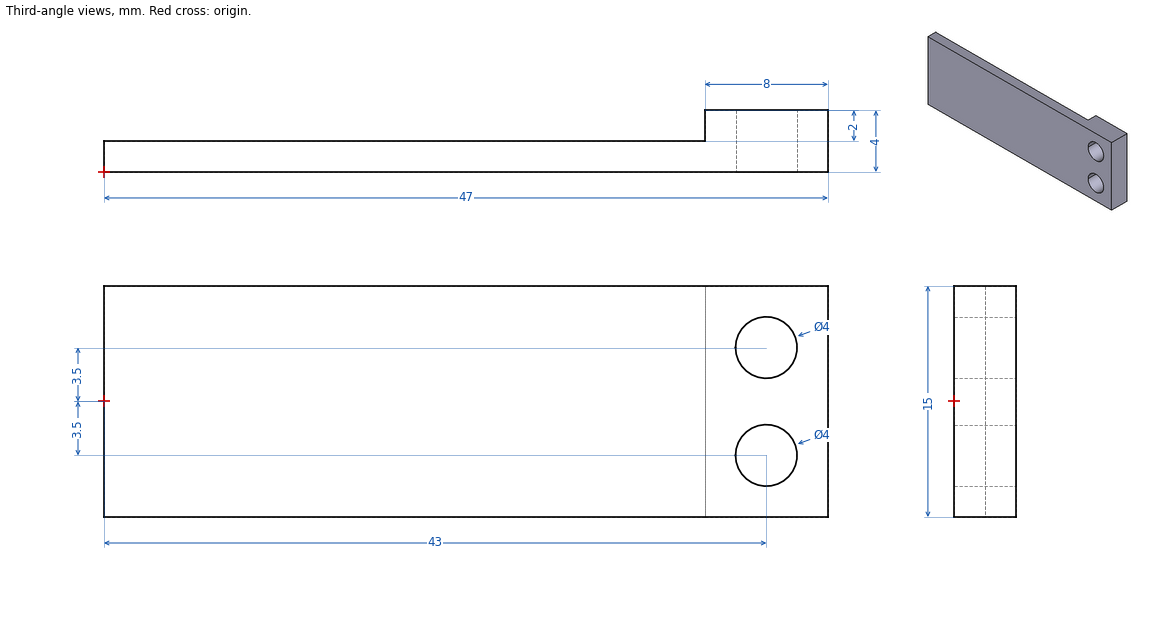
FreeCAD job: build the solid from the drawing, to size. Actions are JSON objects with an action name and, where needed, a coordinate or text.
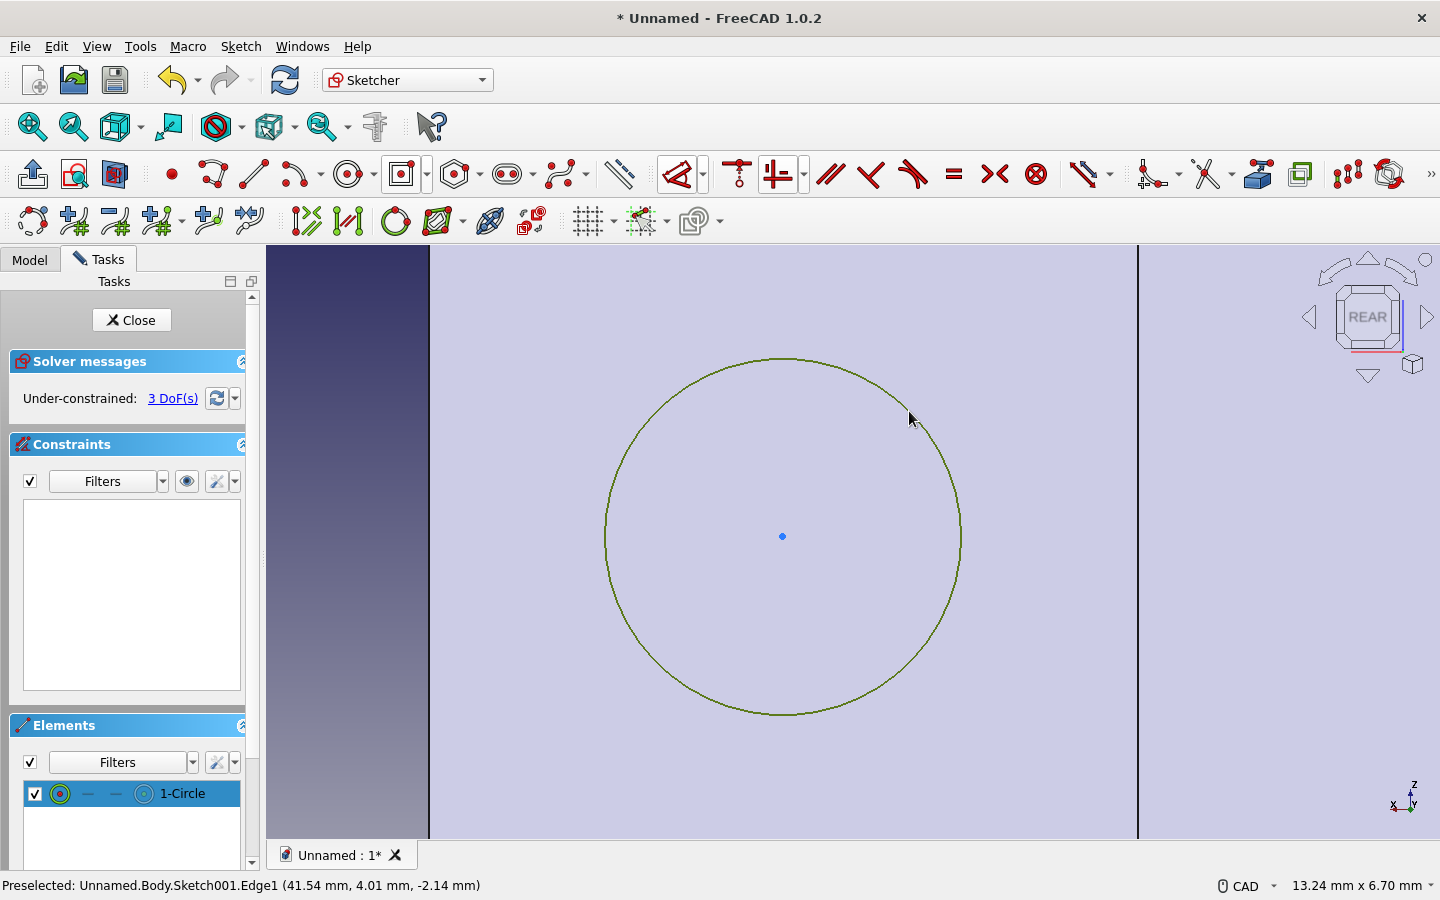
{"action": "left_click", "coordinate": [702, 174]}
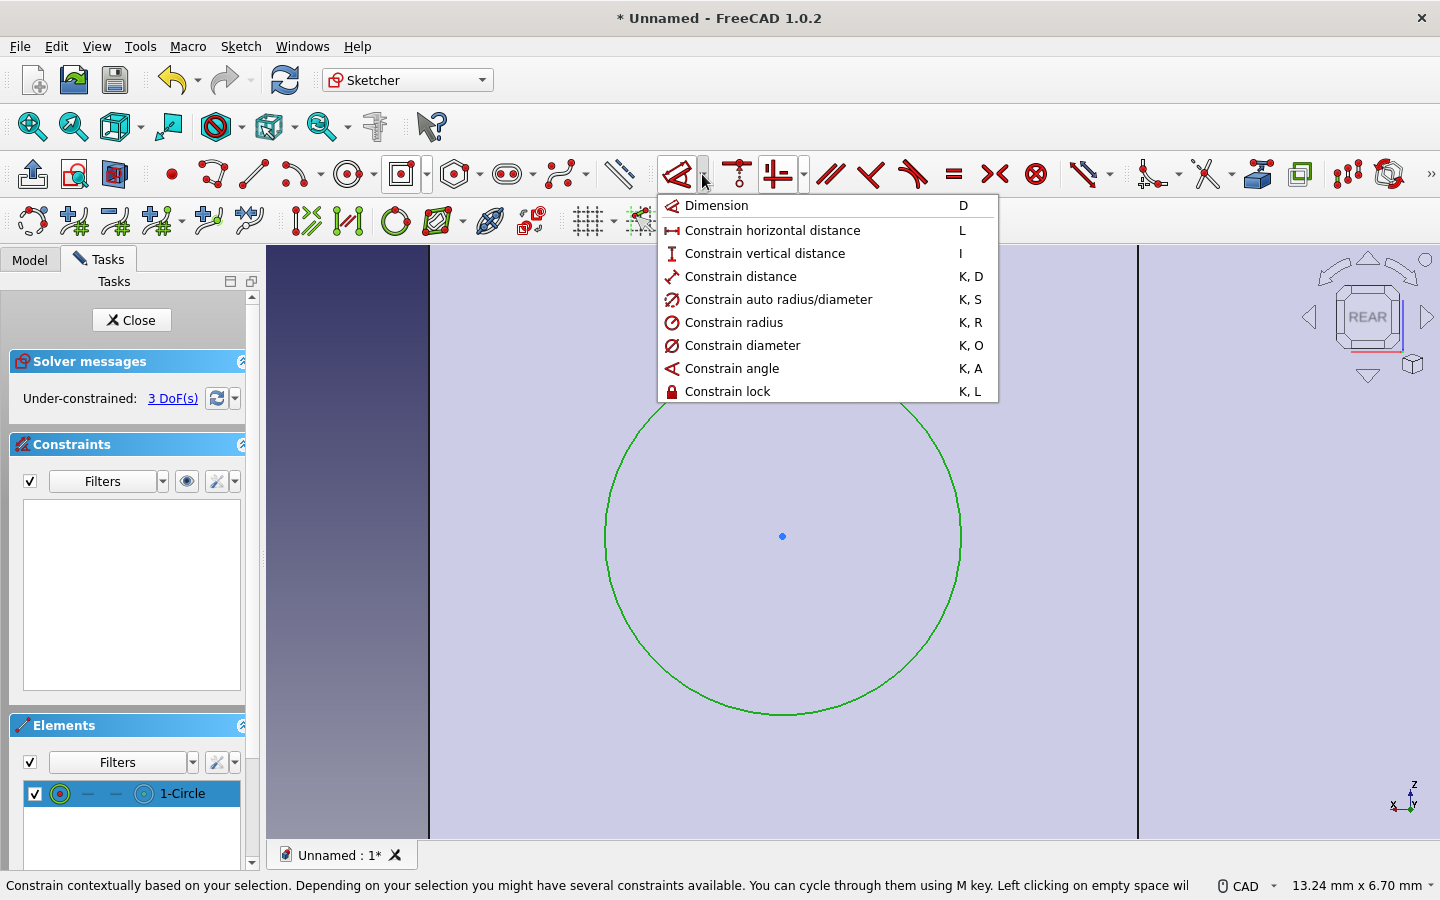
{"action": "left_click", "coordinate": [828, 346]}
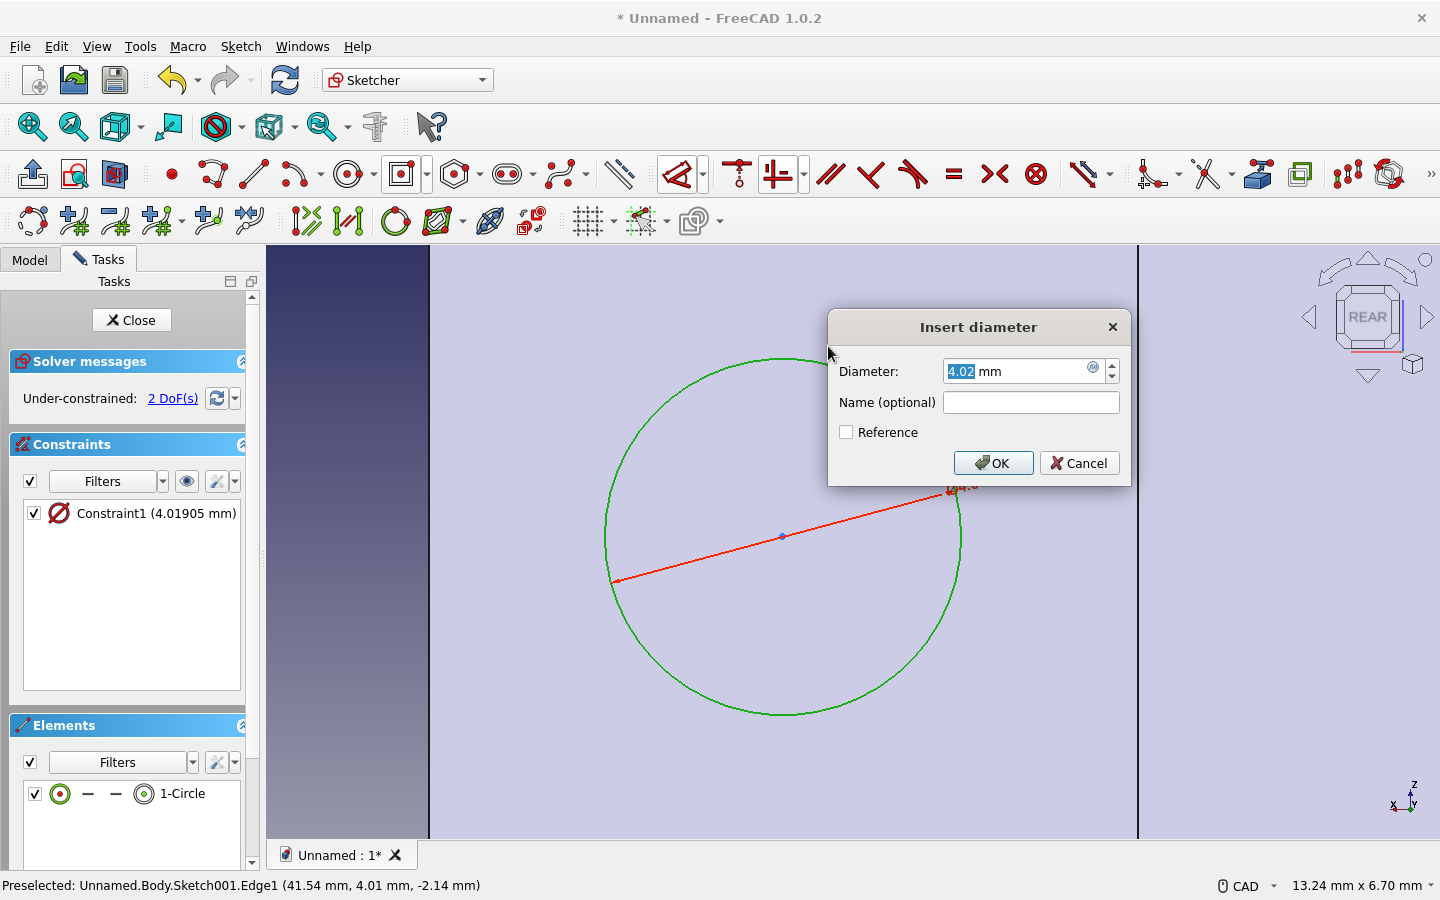
{"action": "type", "text": "4"}
{"action": "key", "text": "Return"}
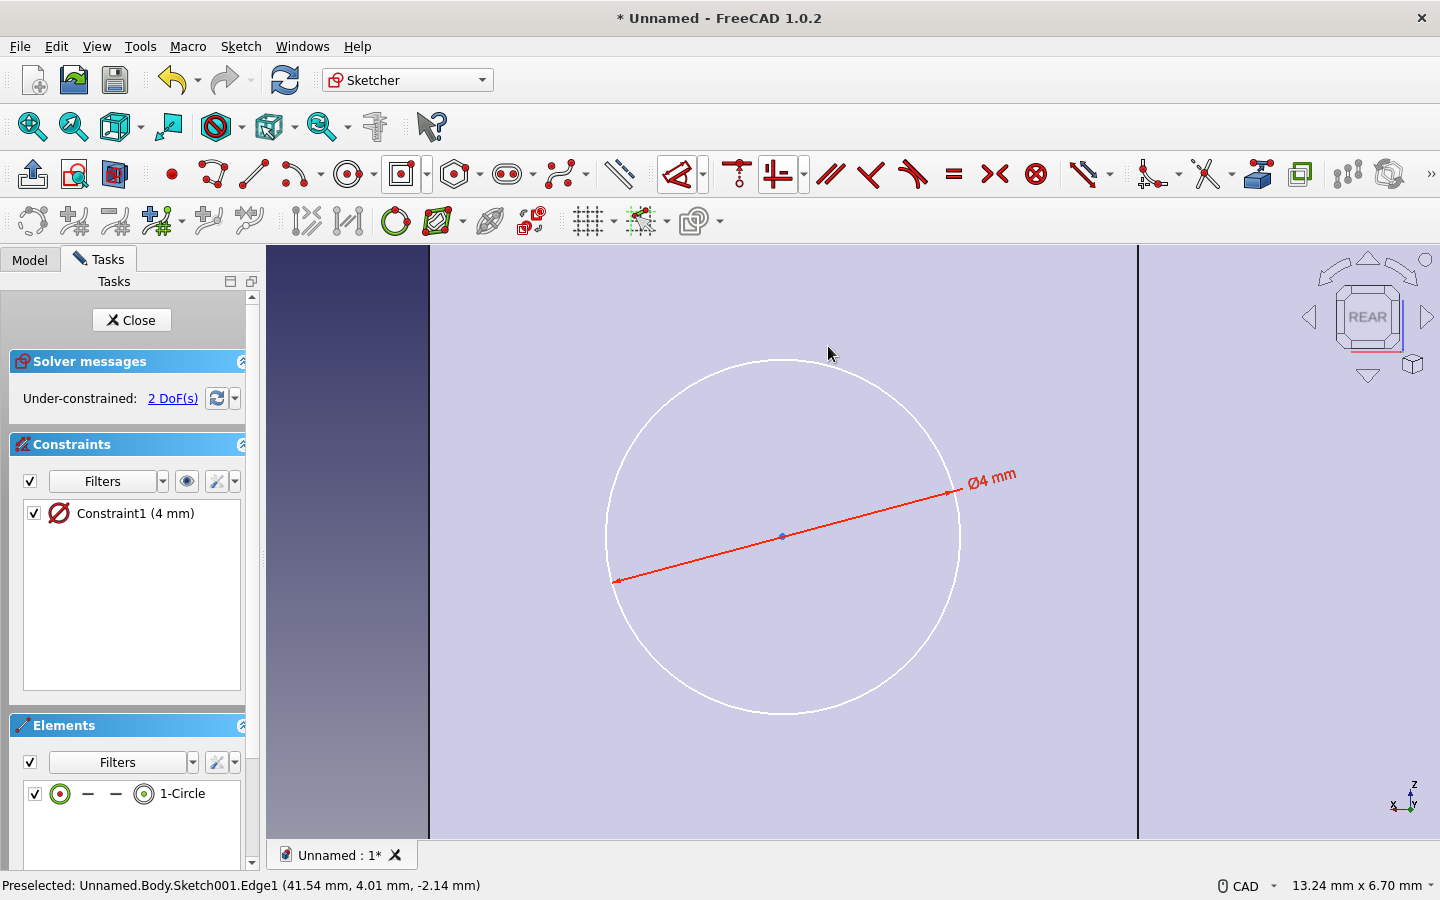
{"action": "left_click", "coordinate": [783, 537]}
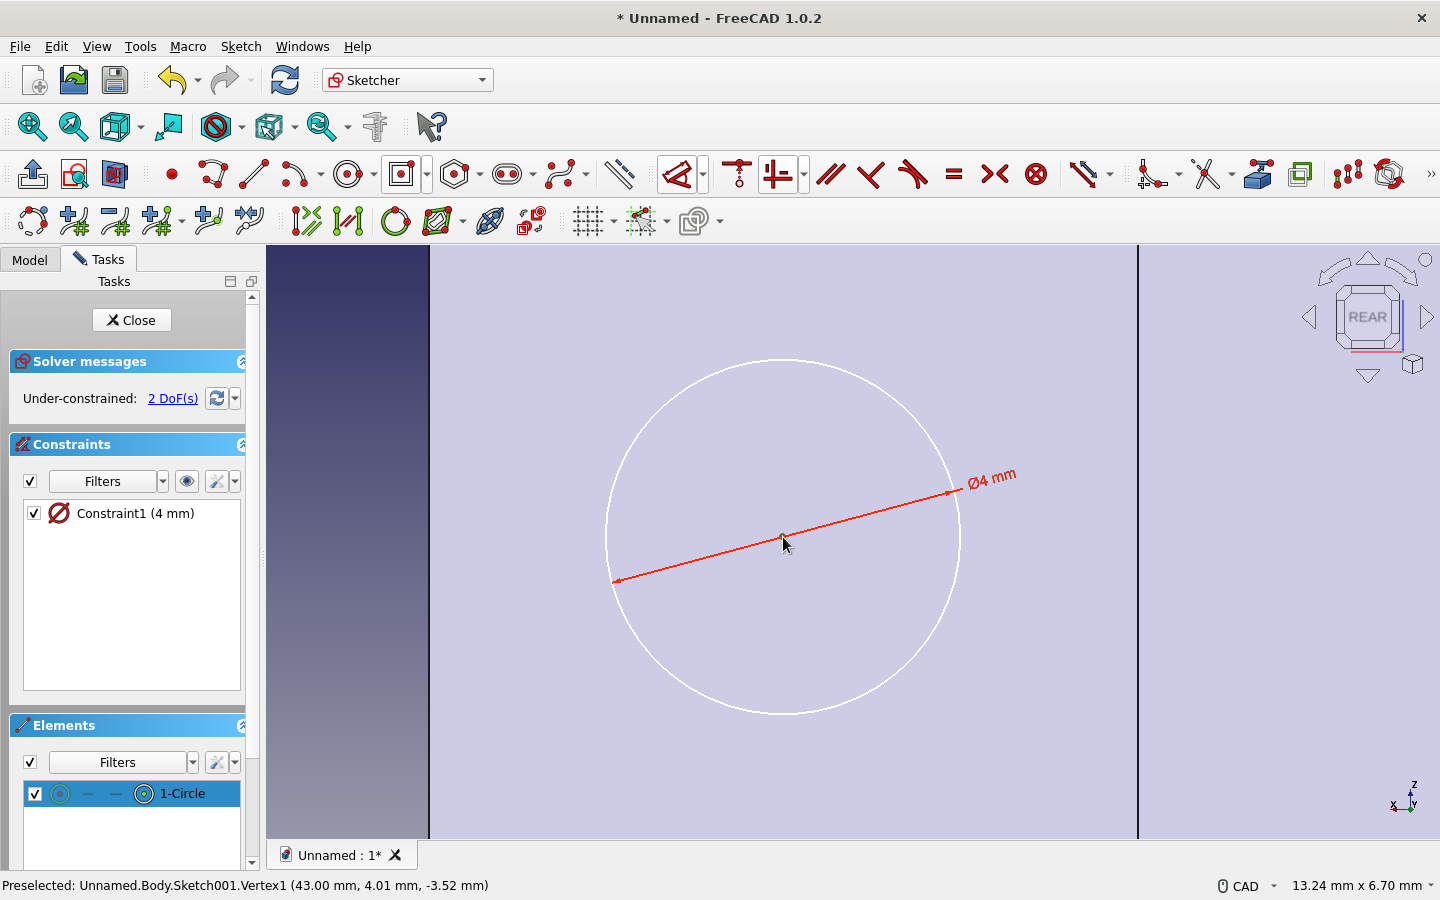
{"action": "left_click", "coordinate": [702, 174]}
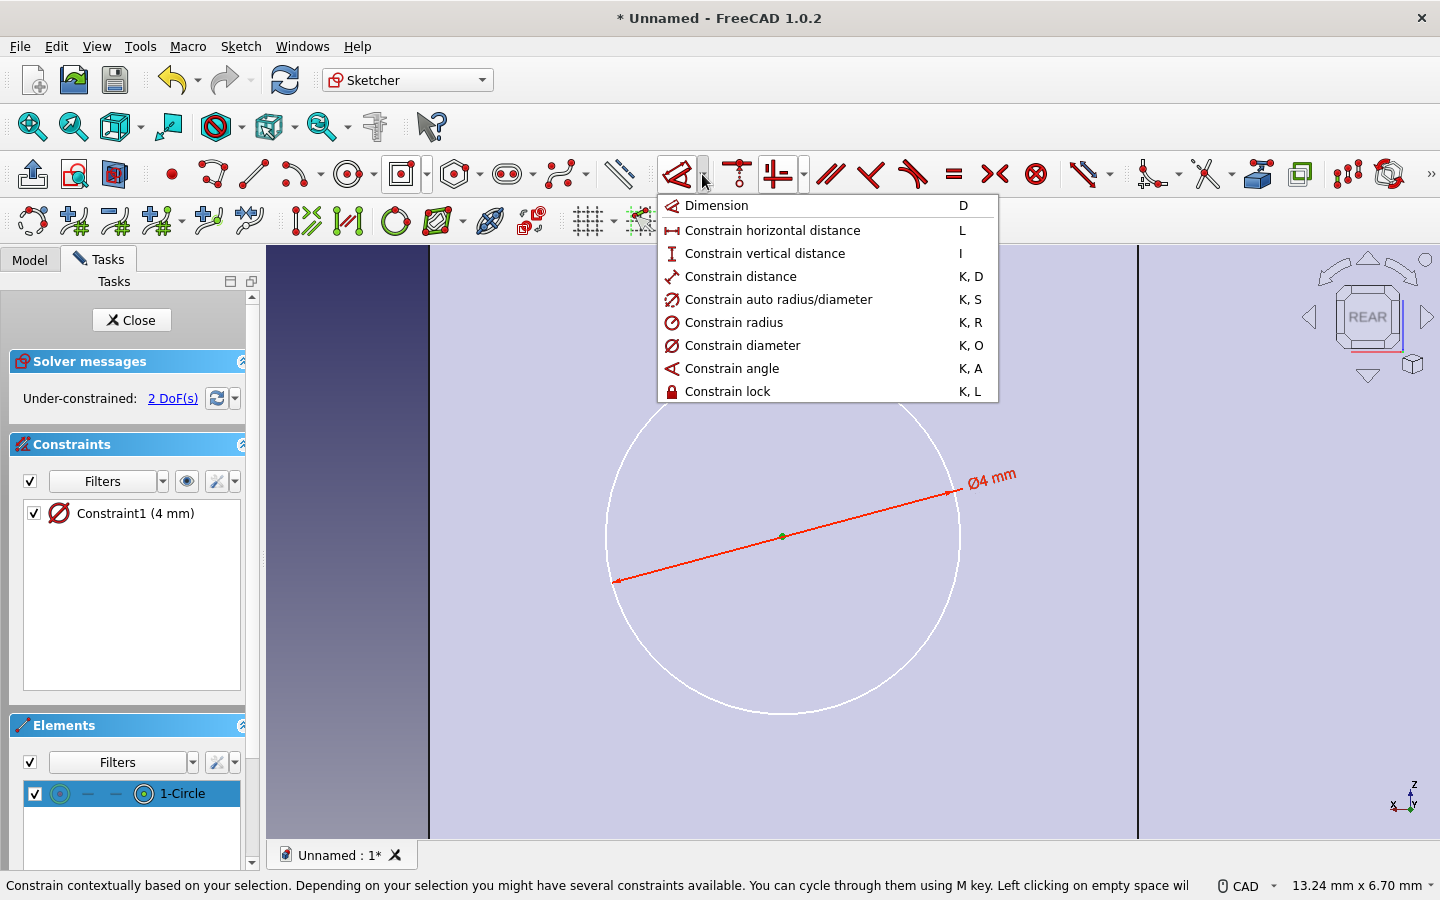
{"action": "left_click", "coordinate": [828, 230]}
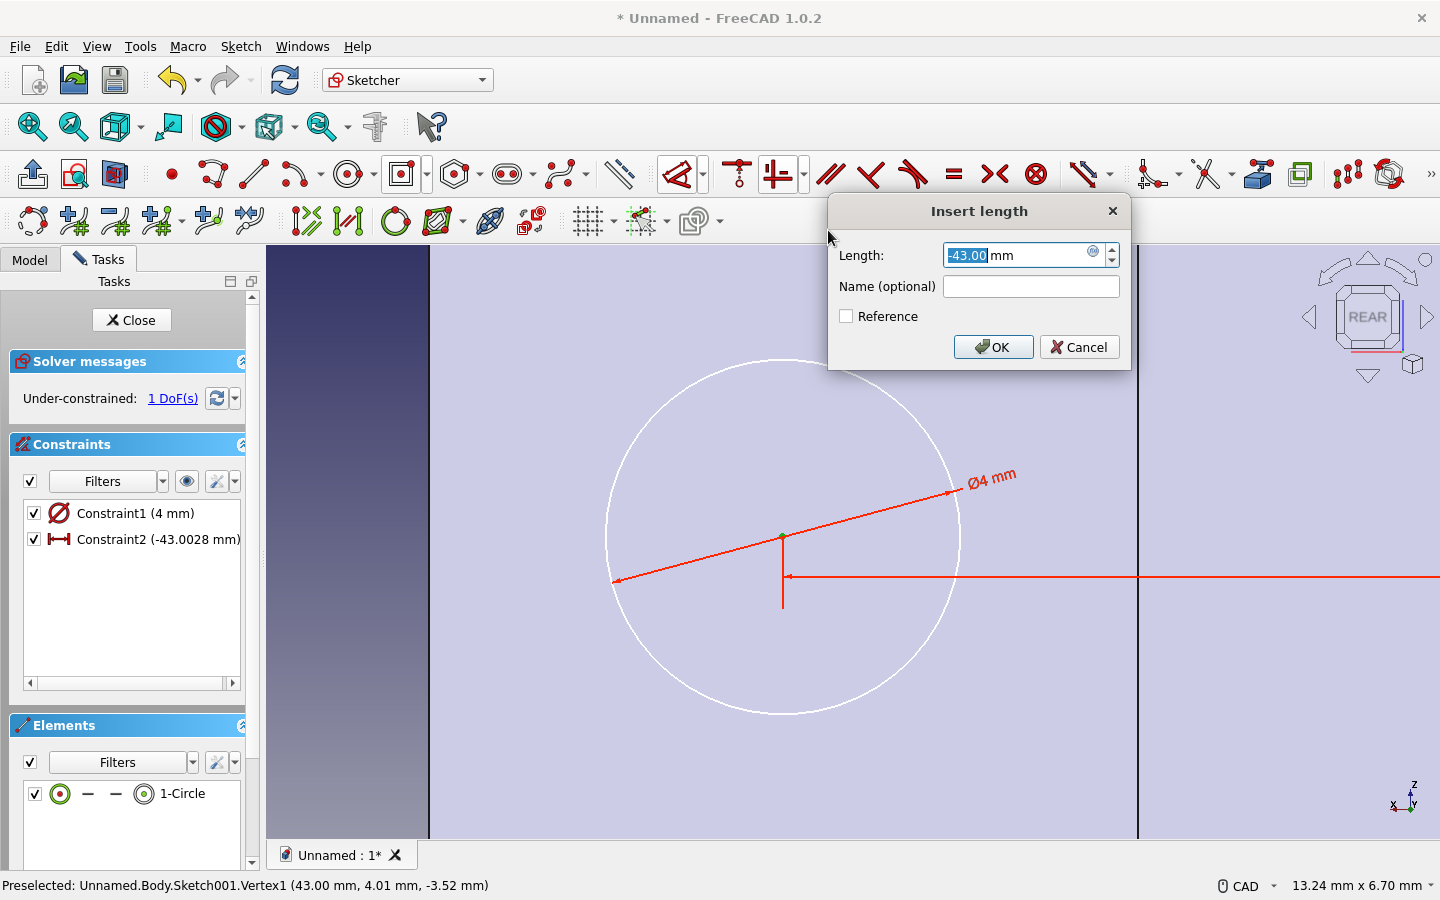
{"action": "type", "text": "-43"}
{"action": "key", "text": "Return"}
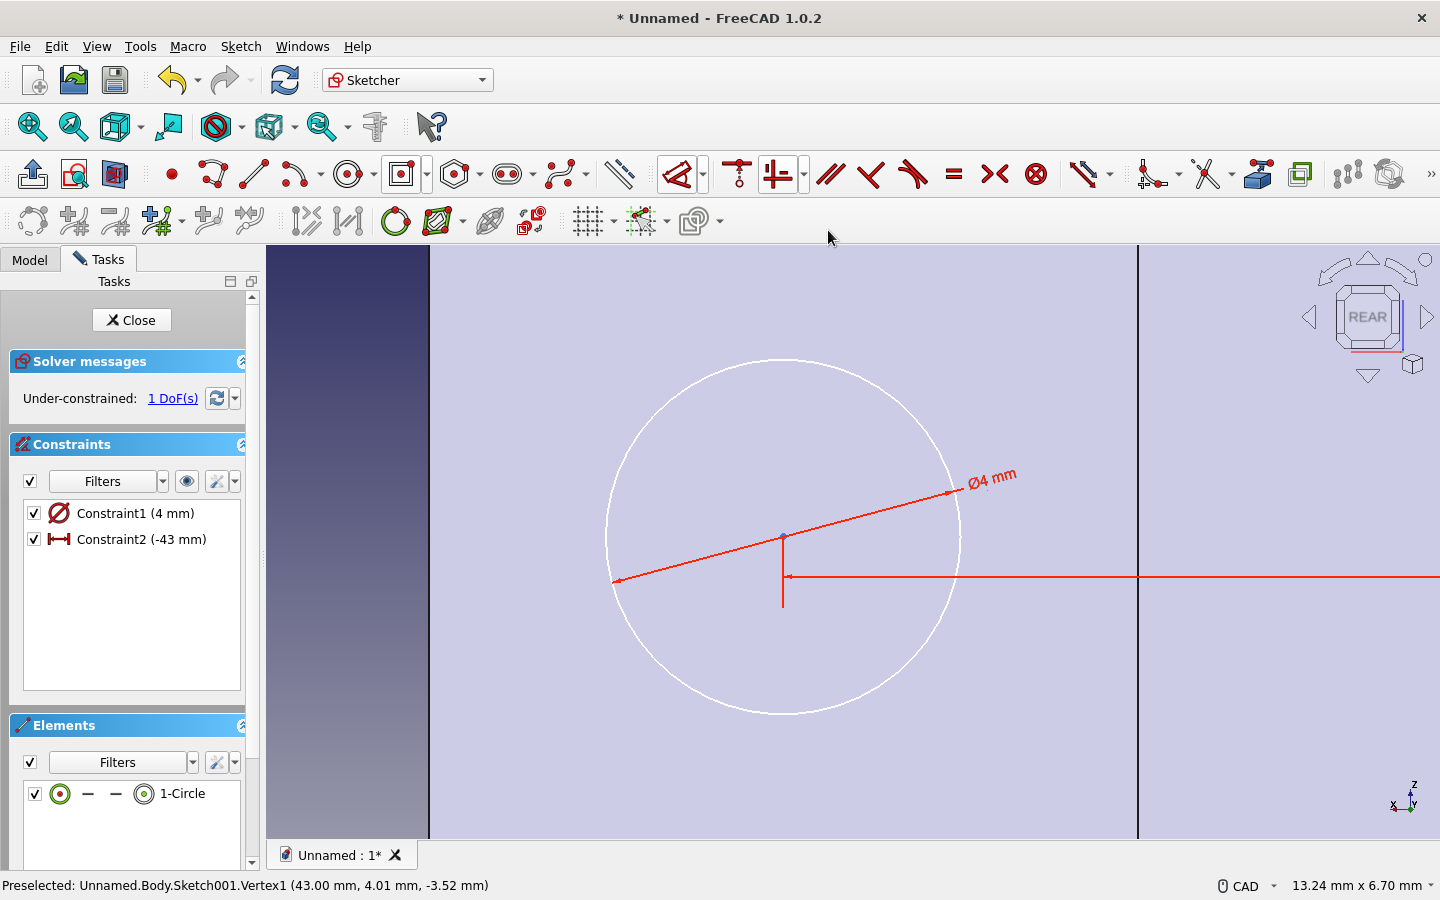
{"action": "left_click", "coordinate": [783, 537]}